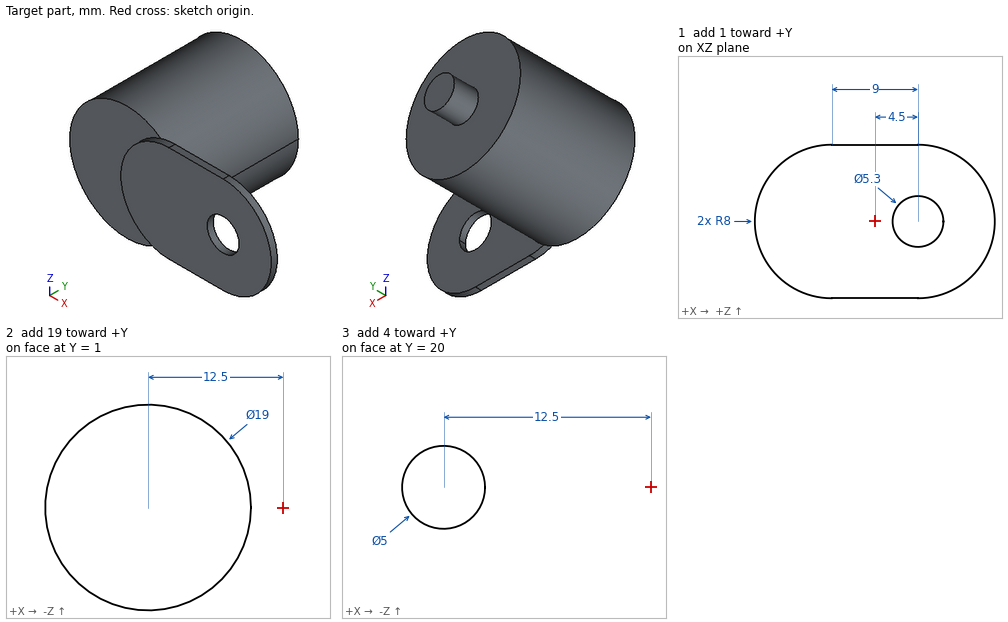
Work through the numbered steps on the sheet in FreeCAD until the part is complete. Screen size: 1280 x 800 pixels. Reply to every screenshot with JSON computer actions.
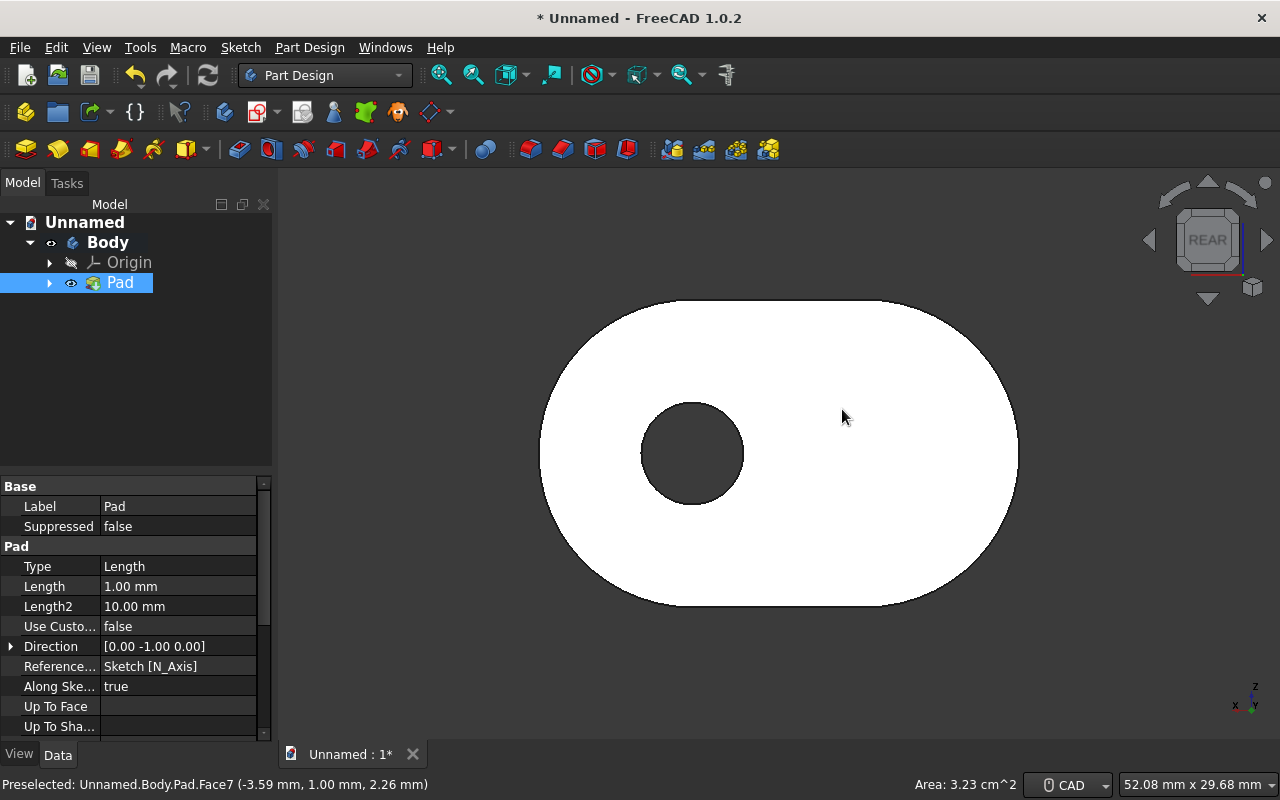
{"action": "left_click", "coordinate": [258, 112]}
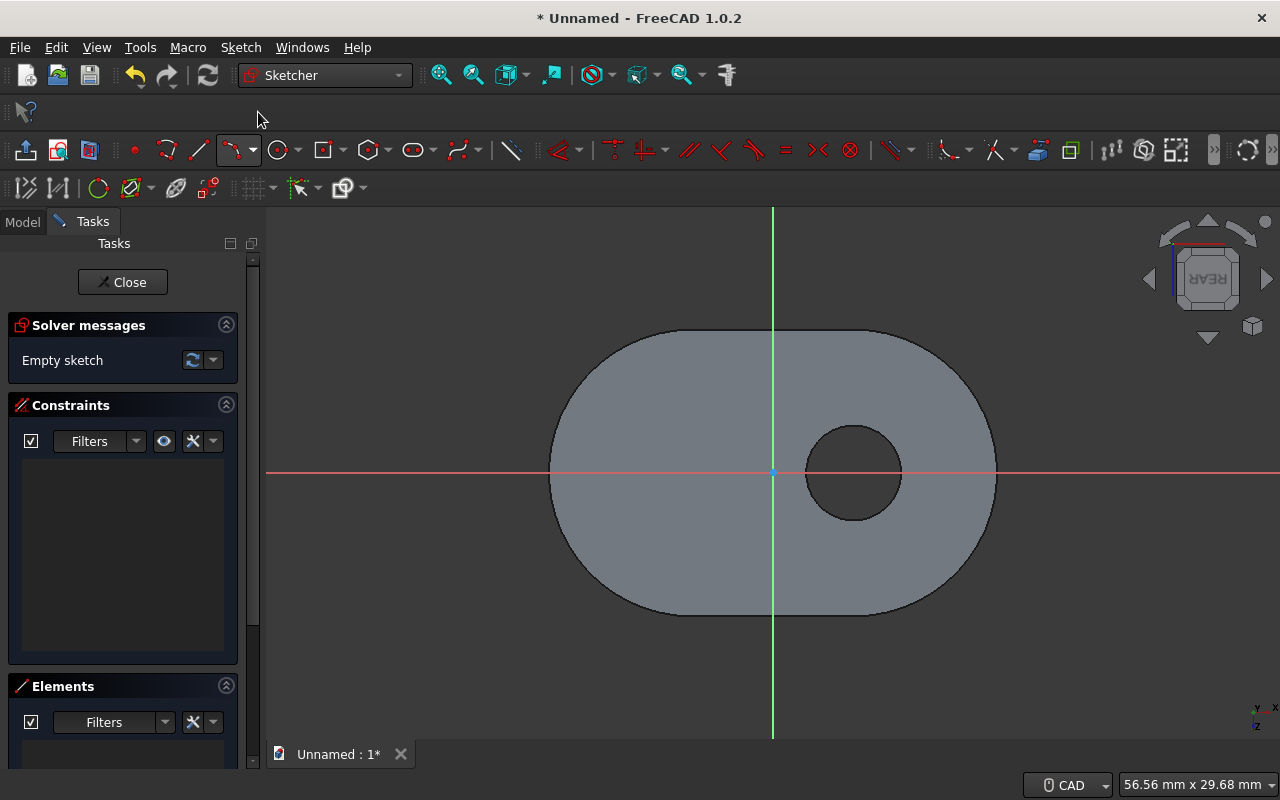
{"action": "left_click", "coordinate": [278, 150]}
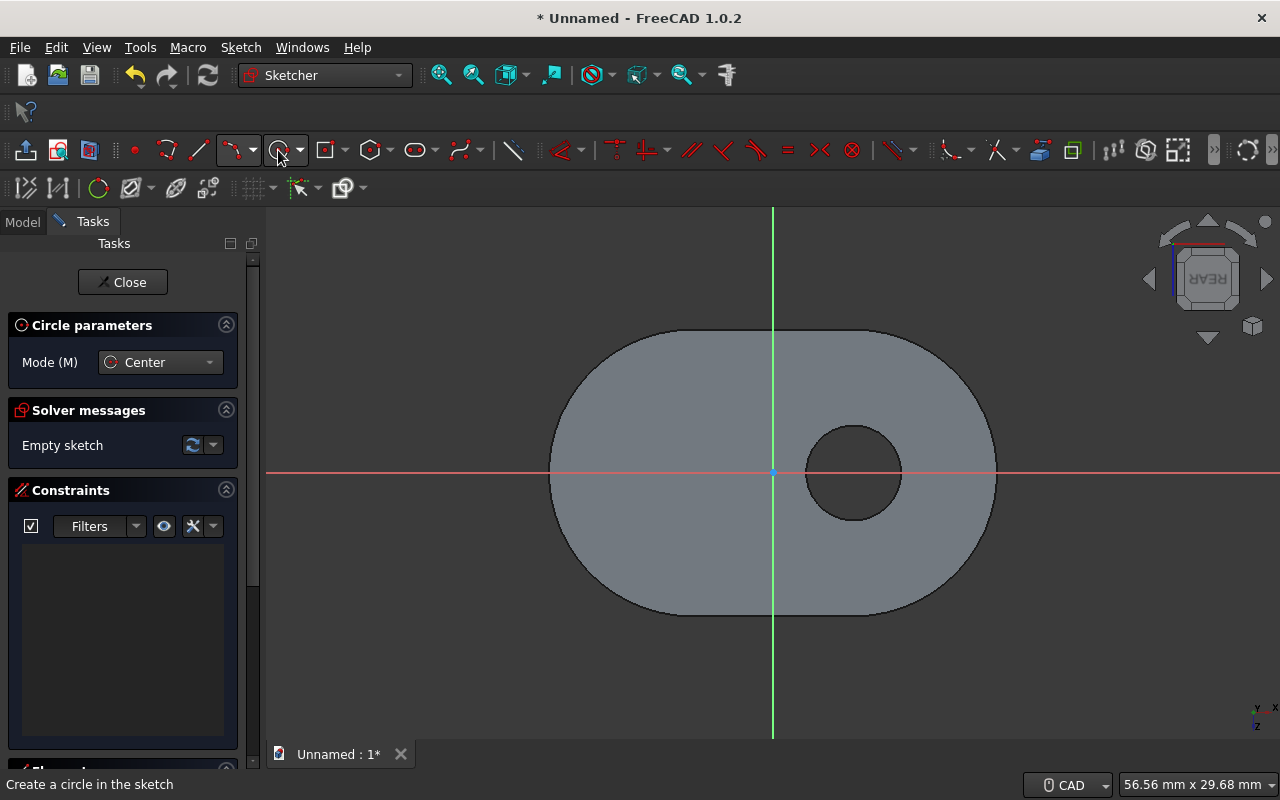
{"action": "left_click", "coordinate": [549, 473]}
{"action": "left_click", "coordinate": [669, 353]}
{"action": "key", "text": "Escape"}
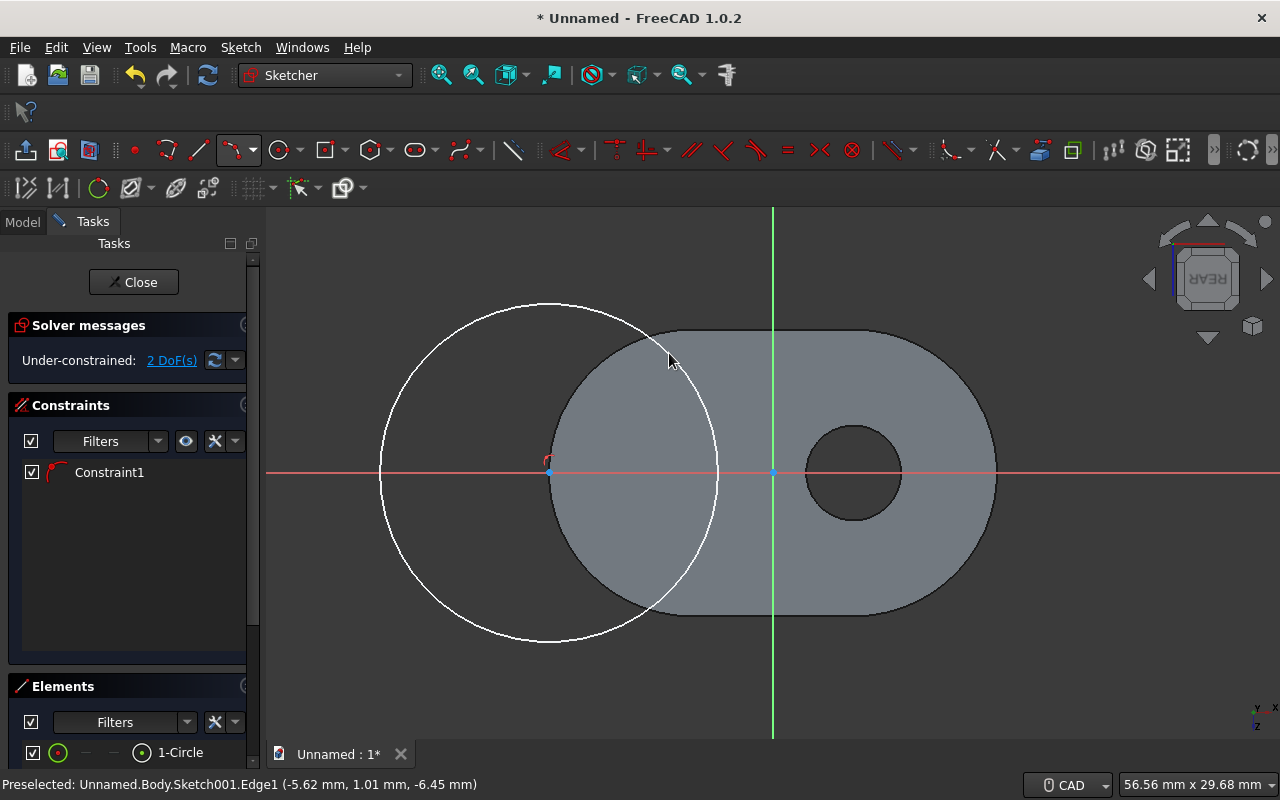
{"action": "left_click", "coordinate": [560, 150]}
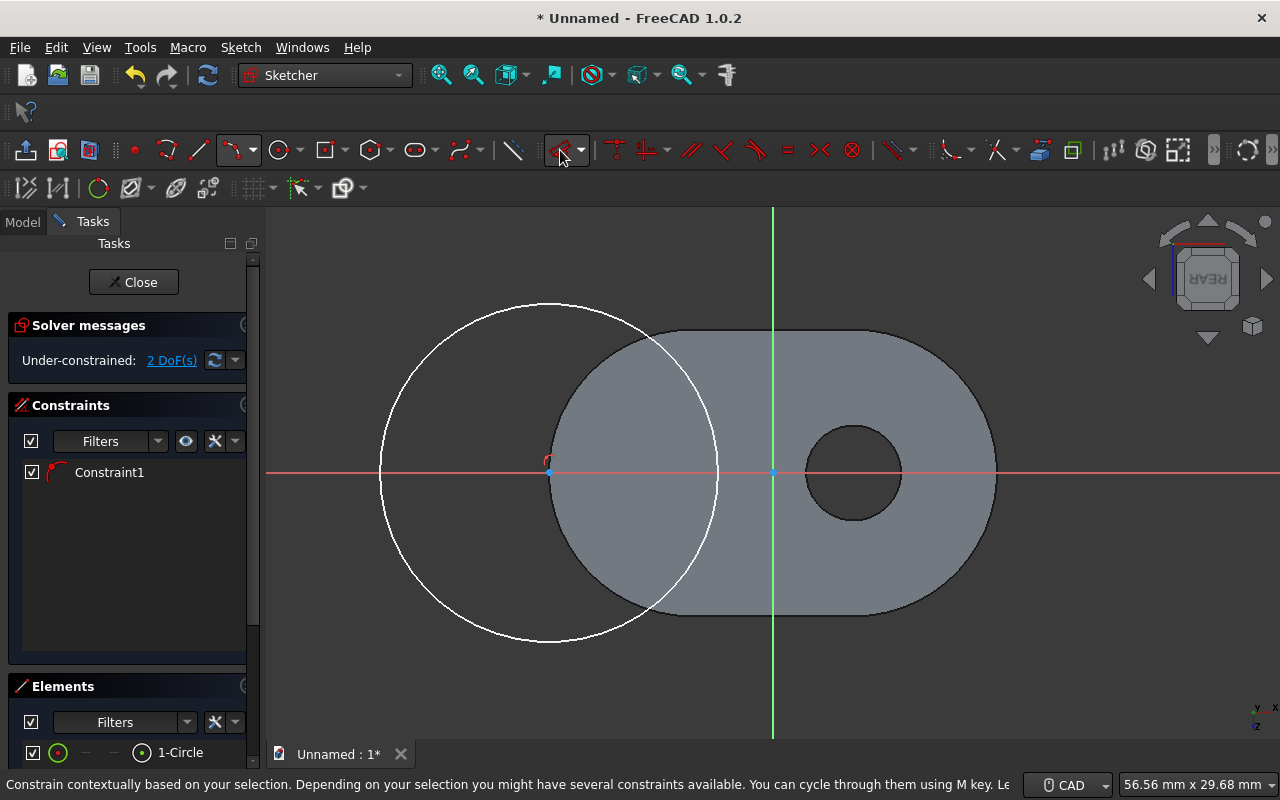
{"action": "left_click", "coordinate": [668, 353]}
{"action": "left_click", "coordinate": [691, 330]}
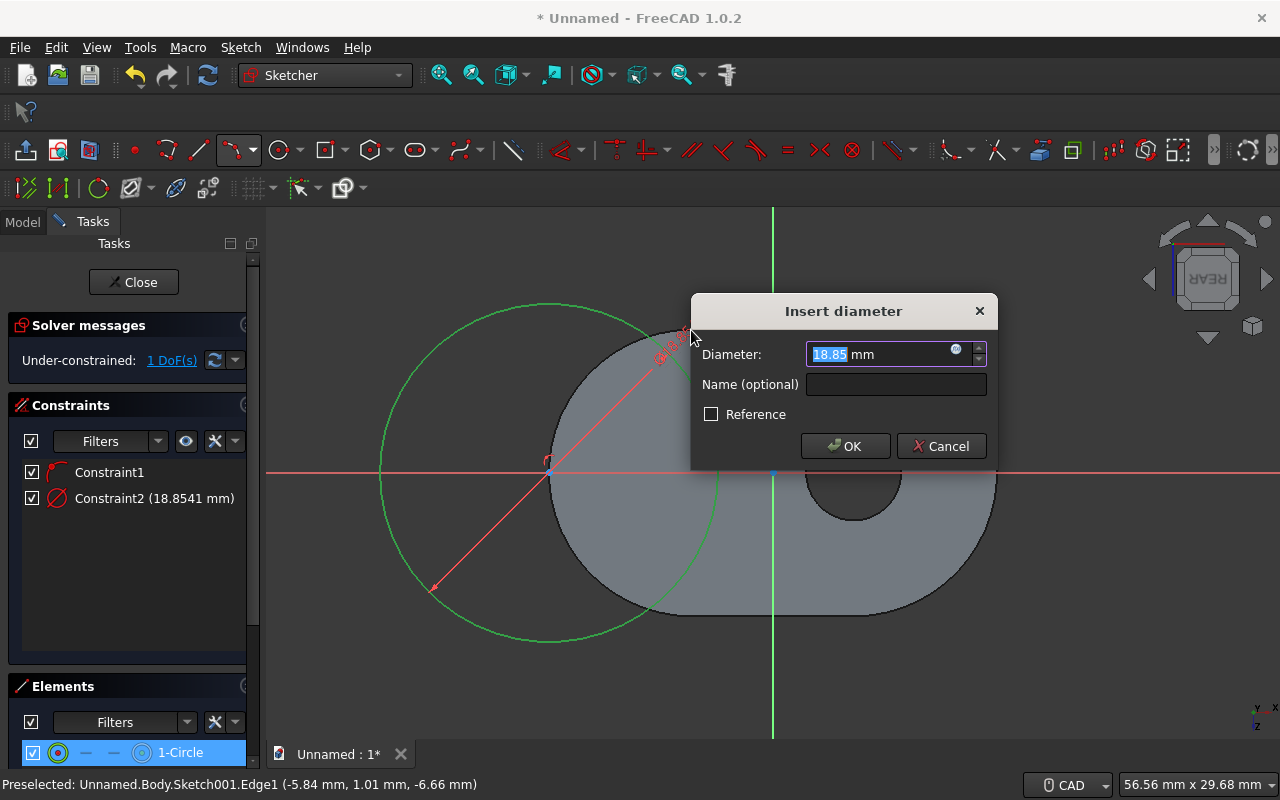
{"action": "type", "text": "19"}
{"action": "key", "text": "Return"}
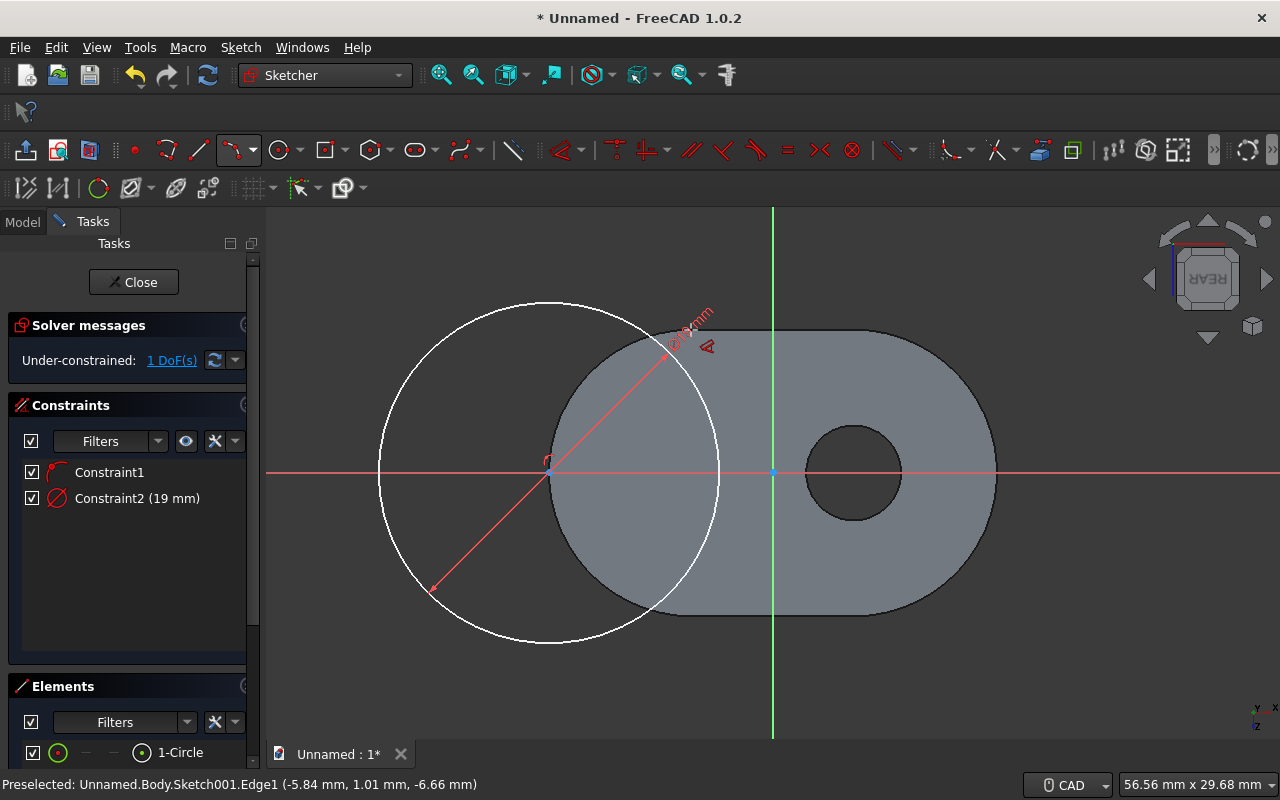
{"action": "left_click", "coordinate": [549, 473]}
{"action": "left_click", "coordinate": [661, 507]}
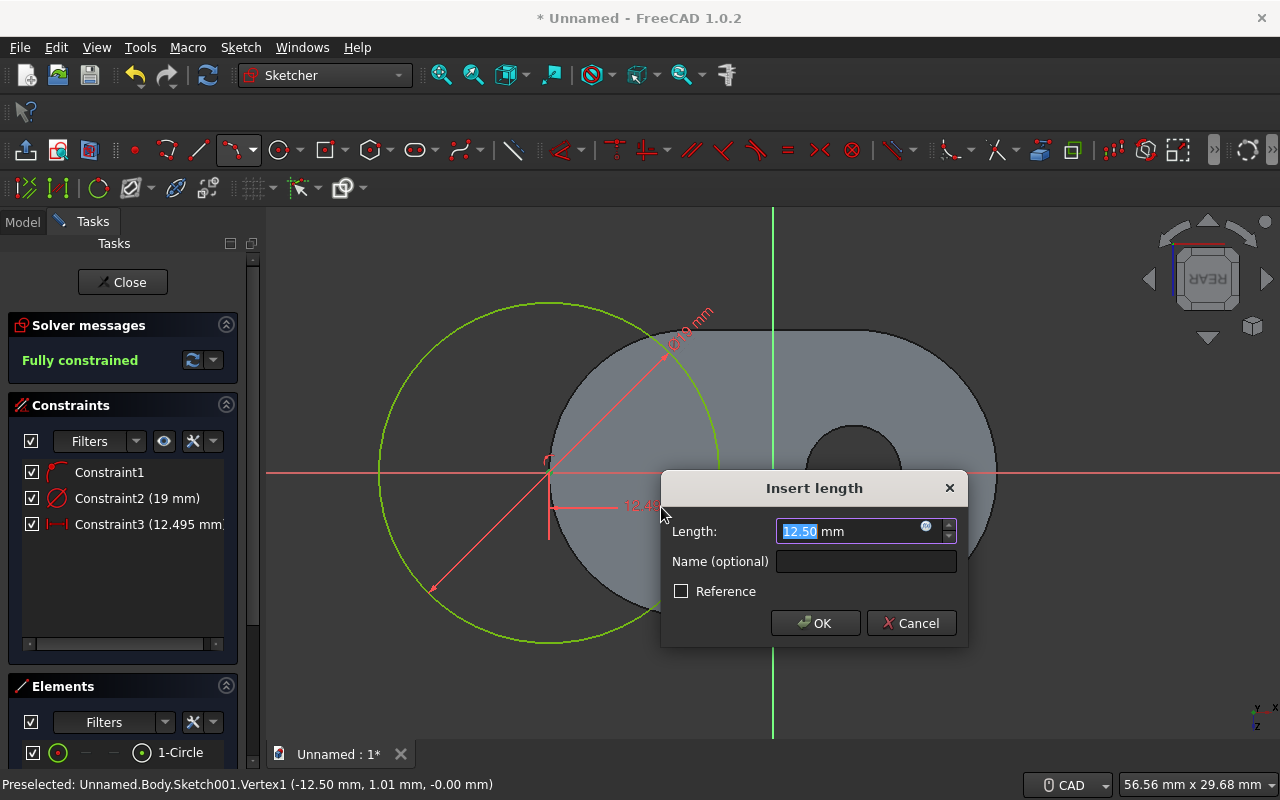
{"action": "type", "text": "12.5"}
{"action": "key", "text": "Return"}
{"action": "key", "text": "Escape"}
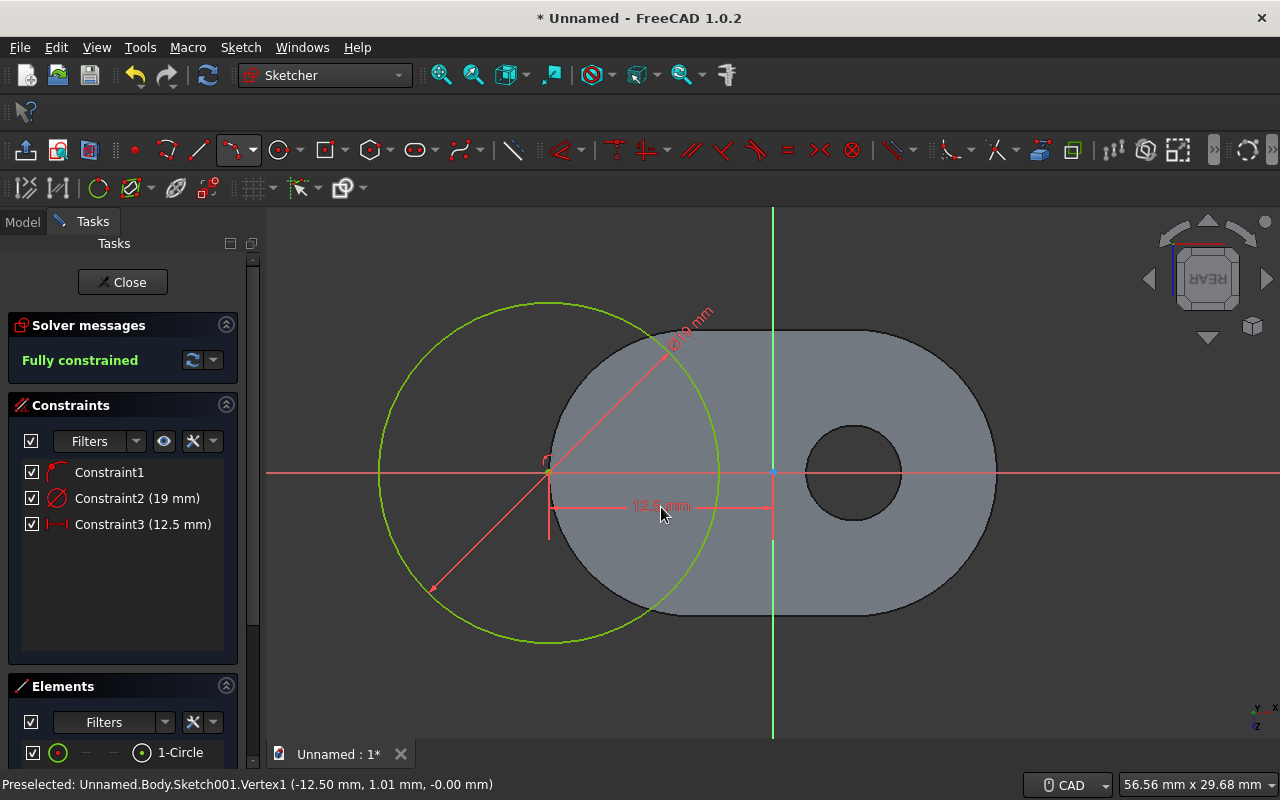
{"action": "left_click", "coordinate": [123, 282]}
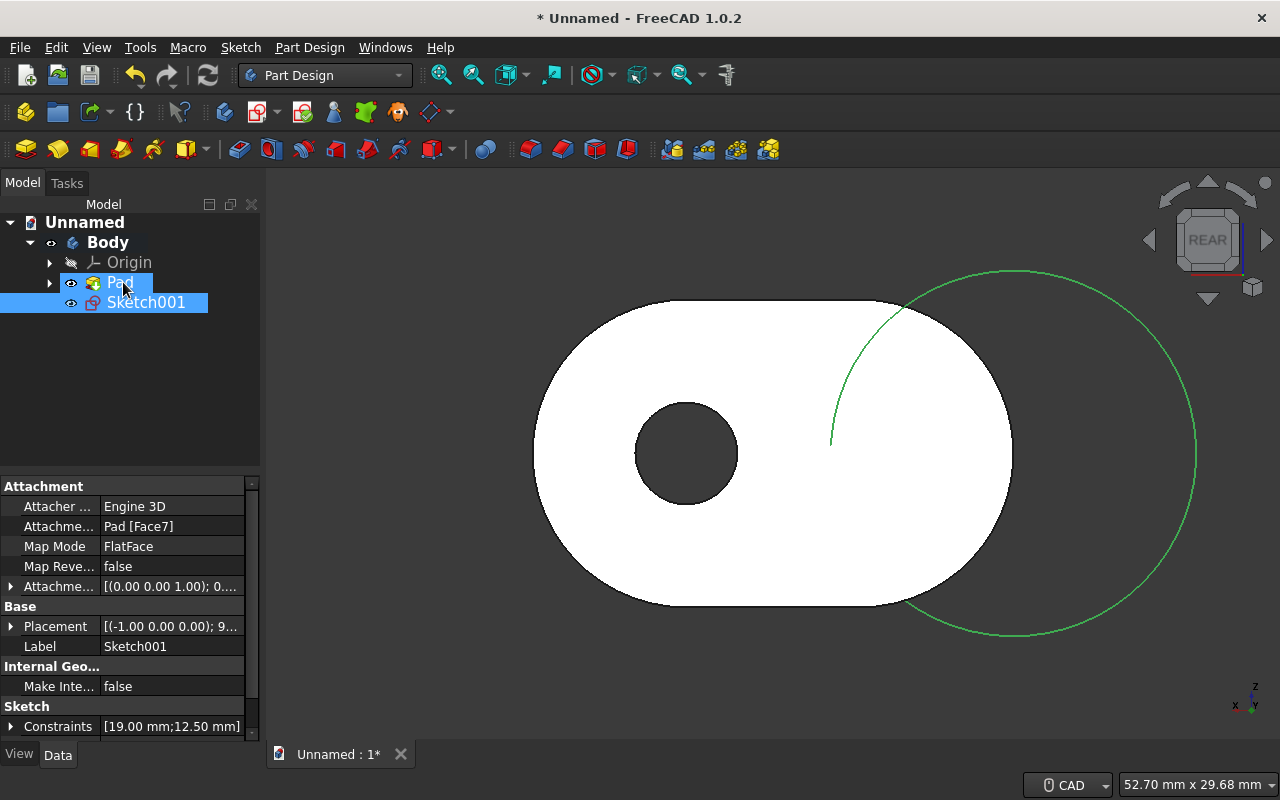
{"action": "left_click", "coordinate": [26, 150]}